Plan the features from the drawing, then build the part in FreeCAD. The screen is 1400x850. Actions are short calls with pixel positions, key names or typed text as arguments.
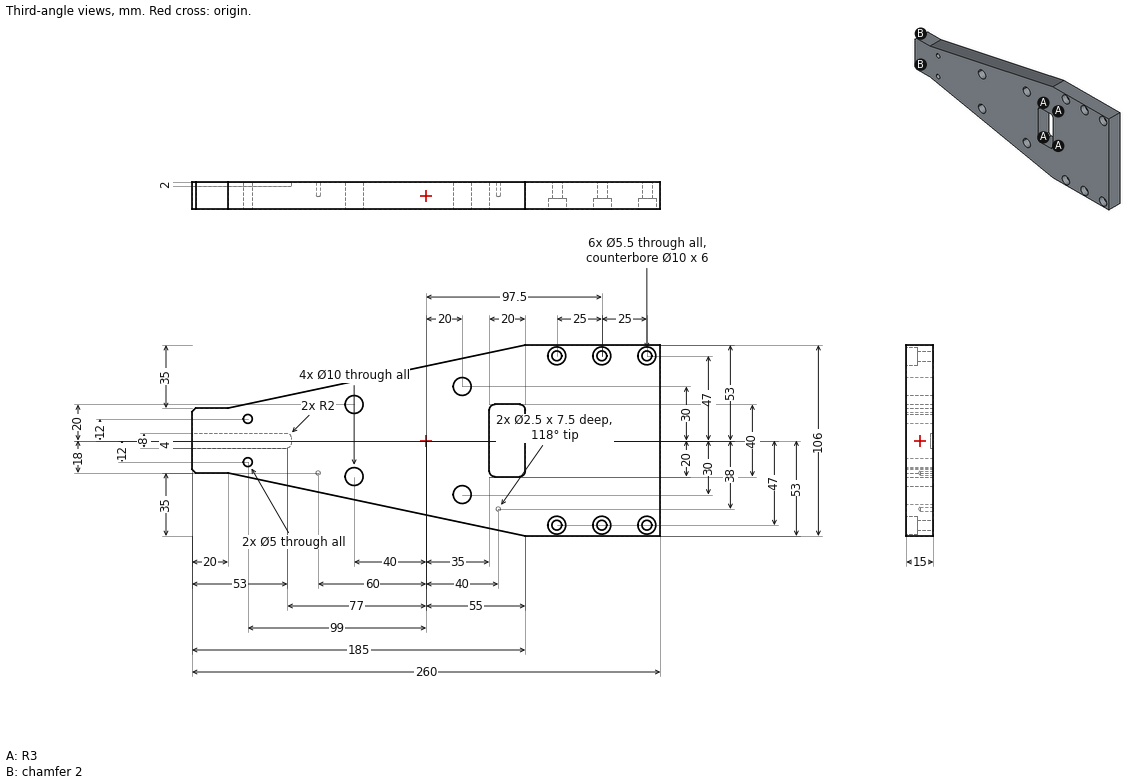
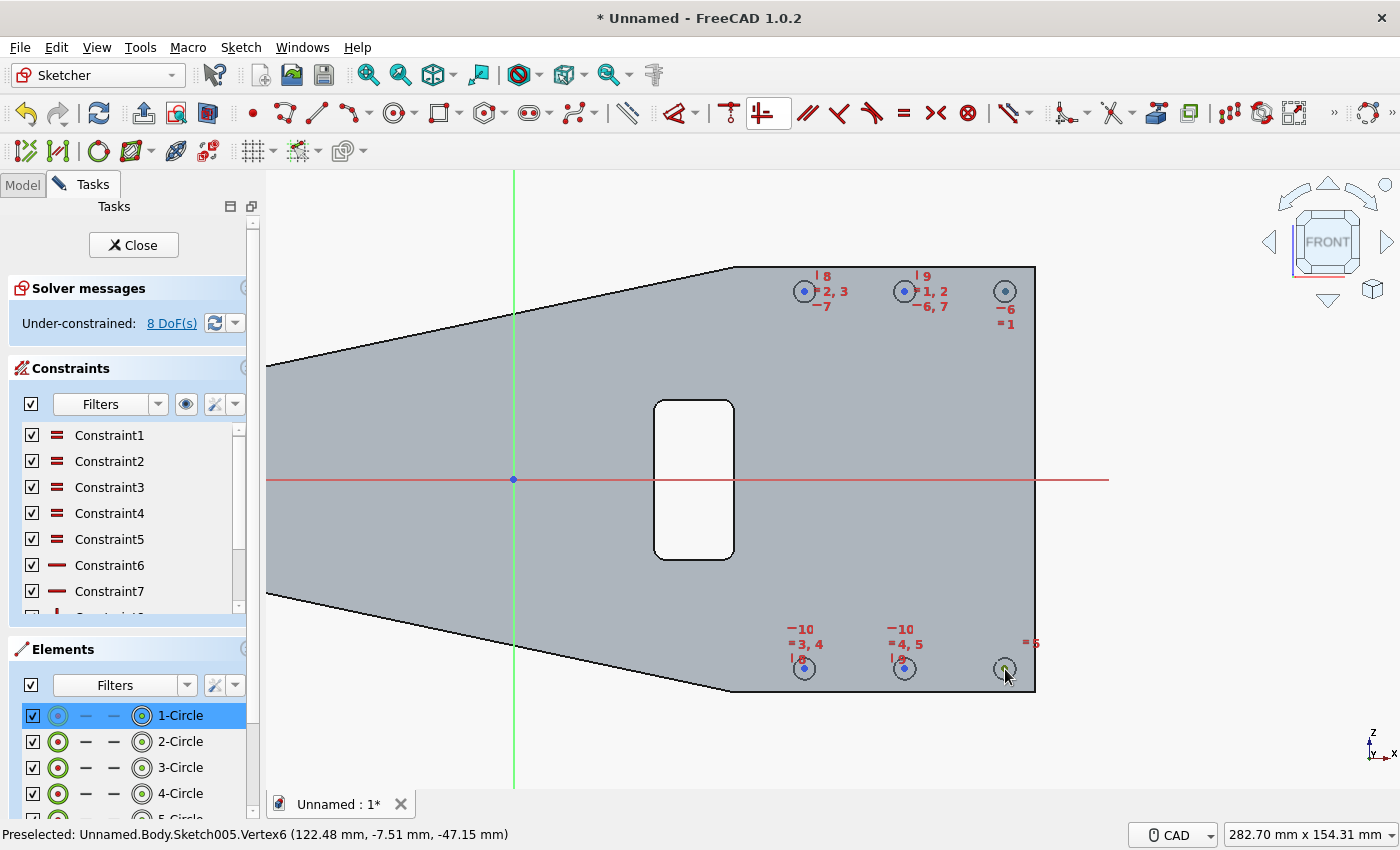
key(v)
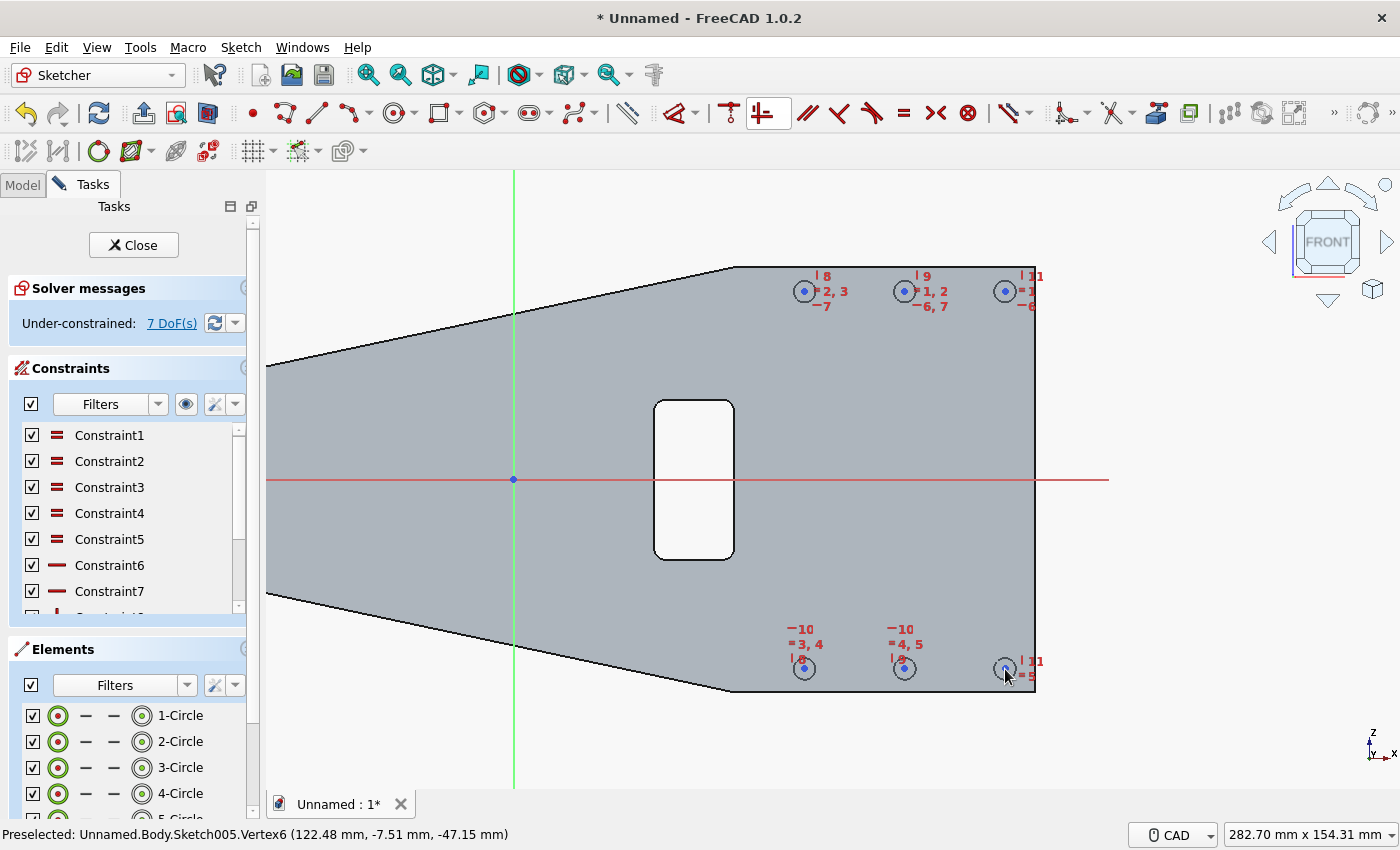
click(905, 669)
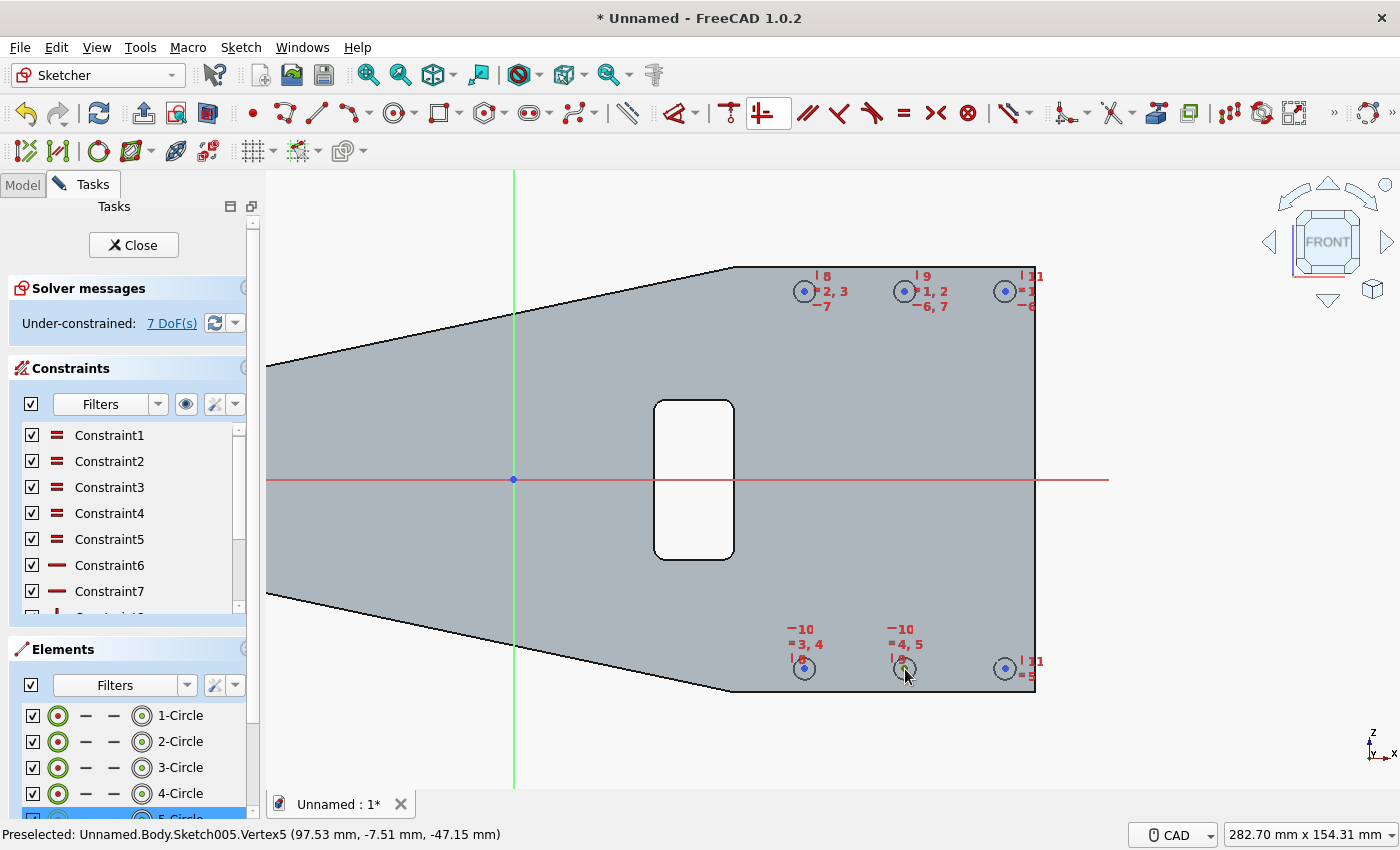
click(1005, 669)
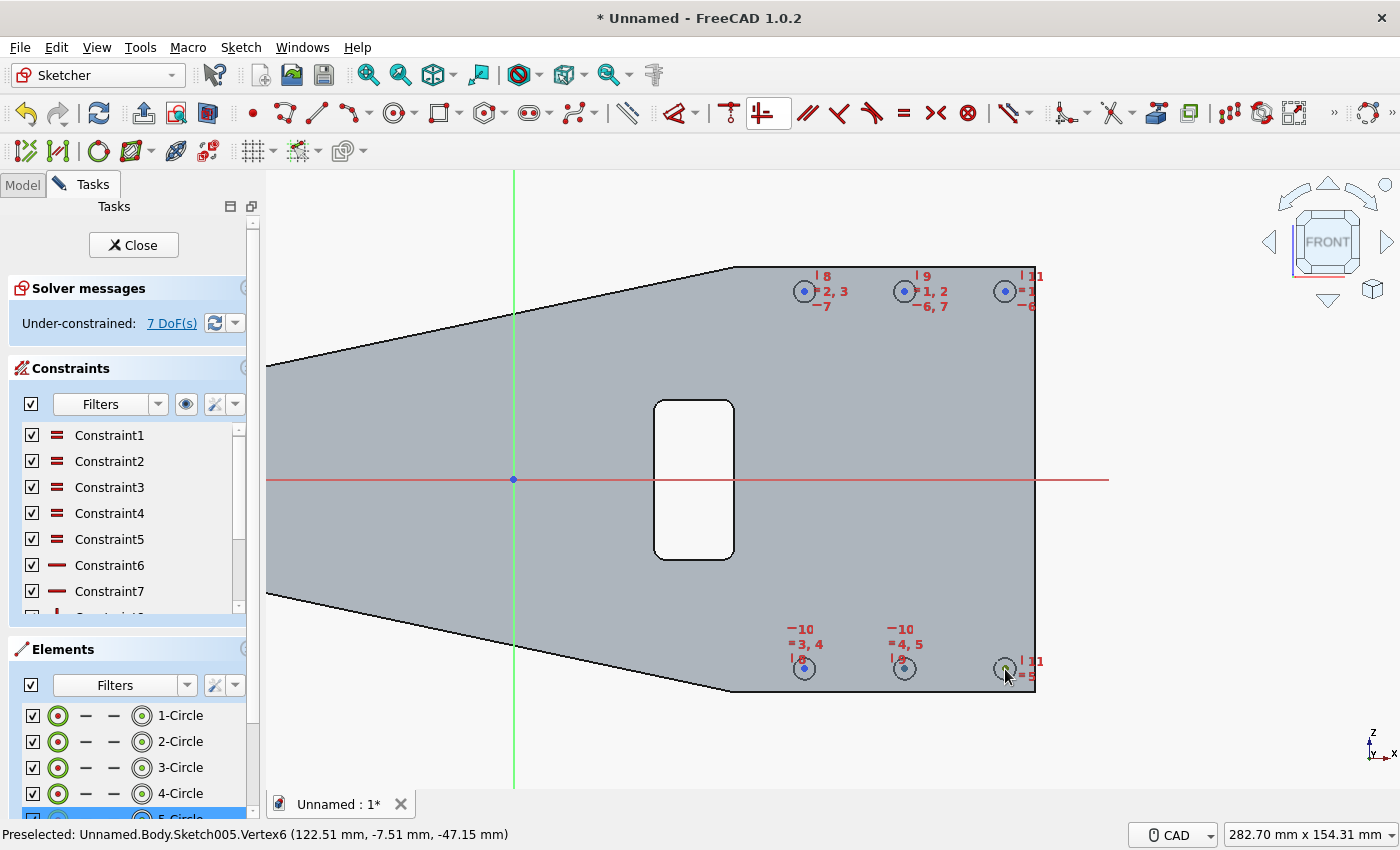
key(h)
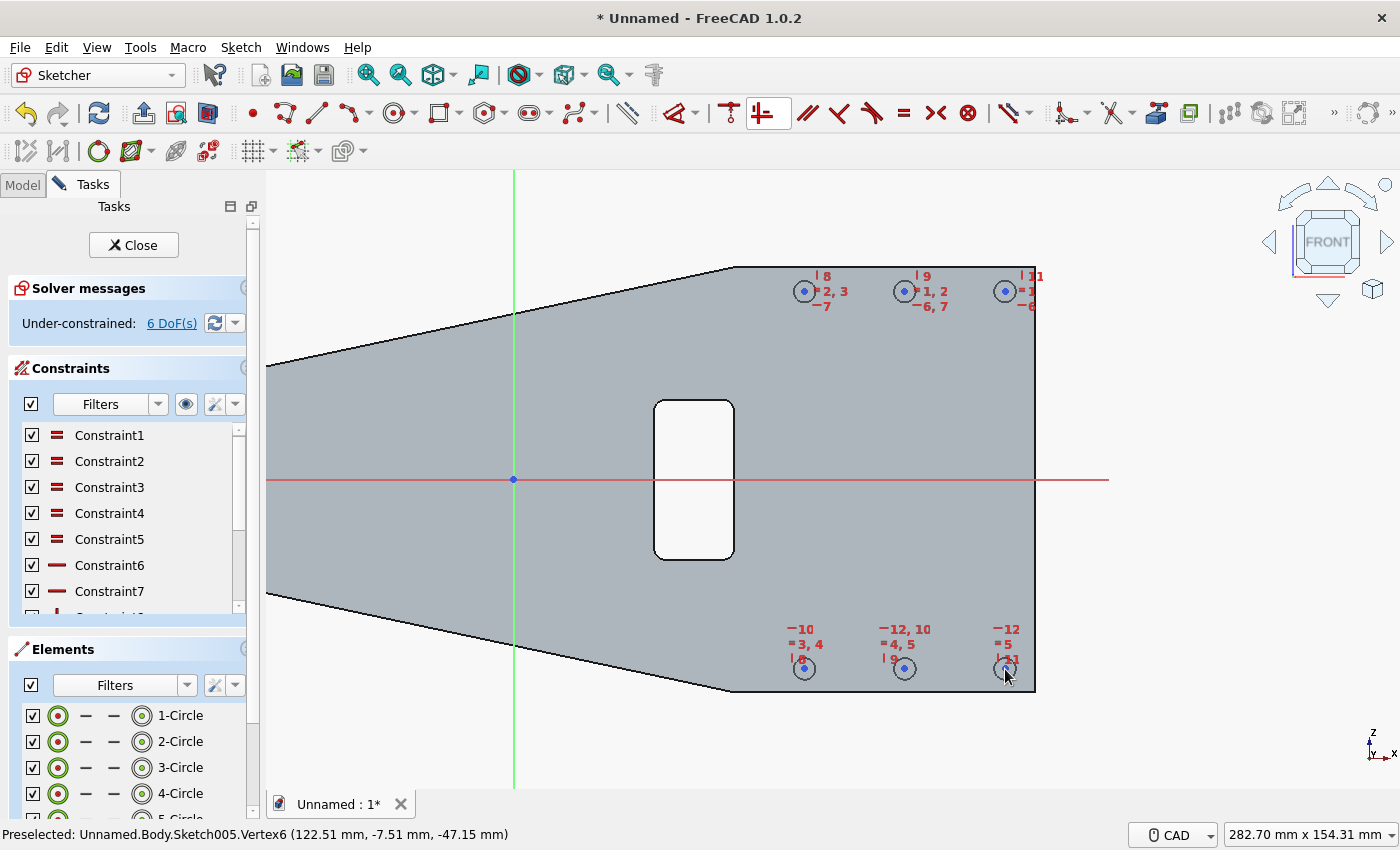
click(674, 114)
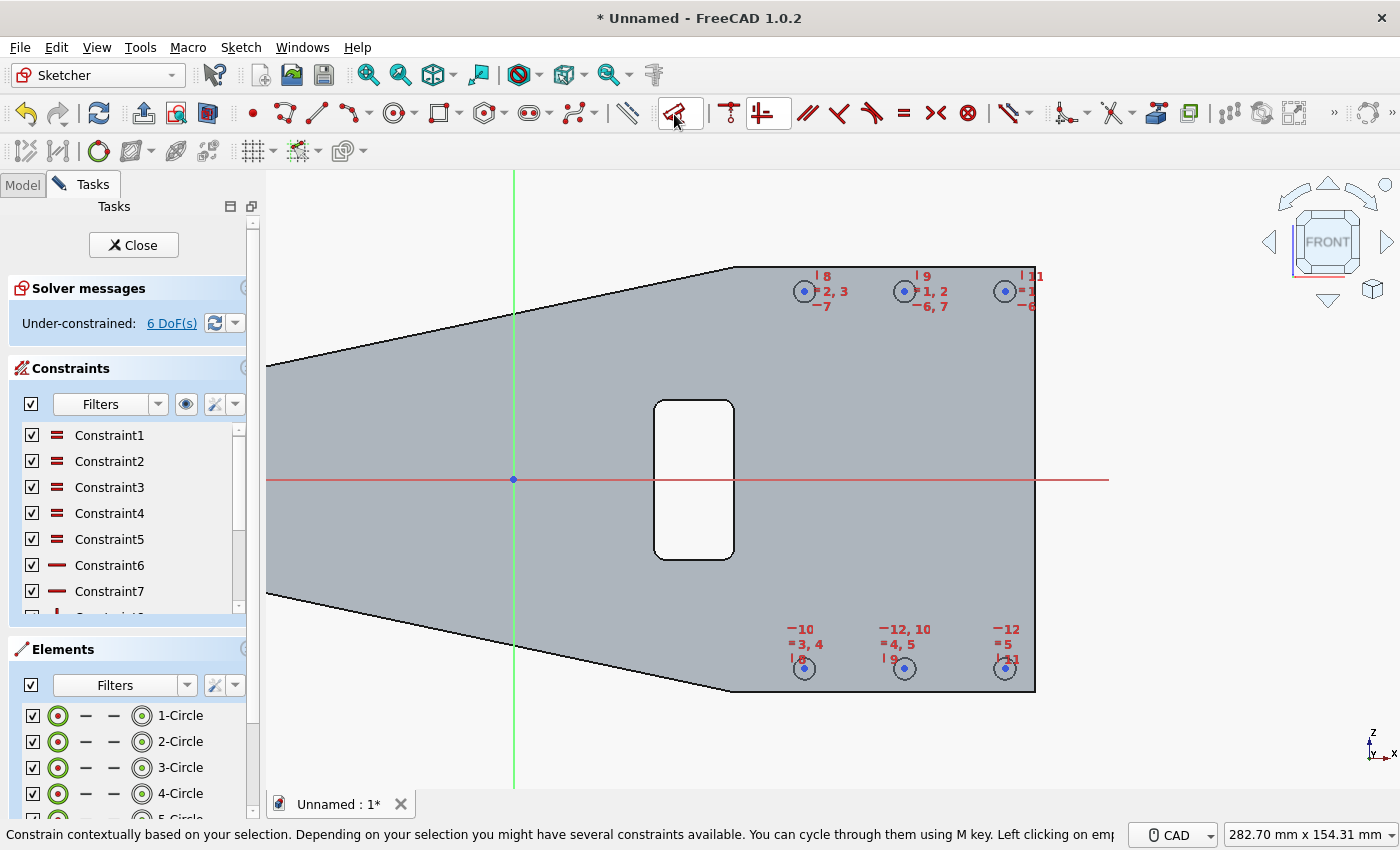
scroll(1013, 284, up, 3)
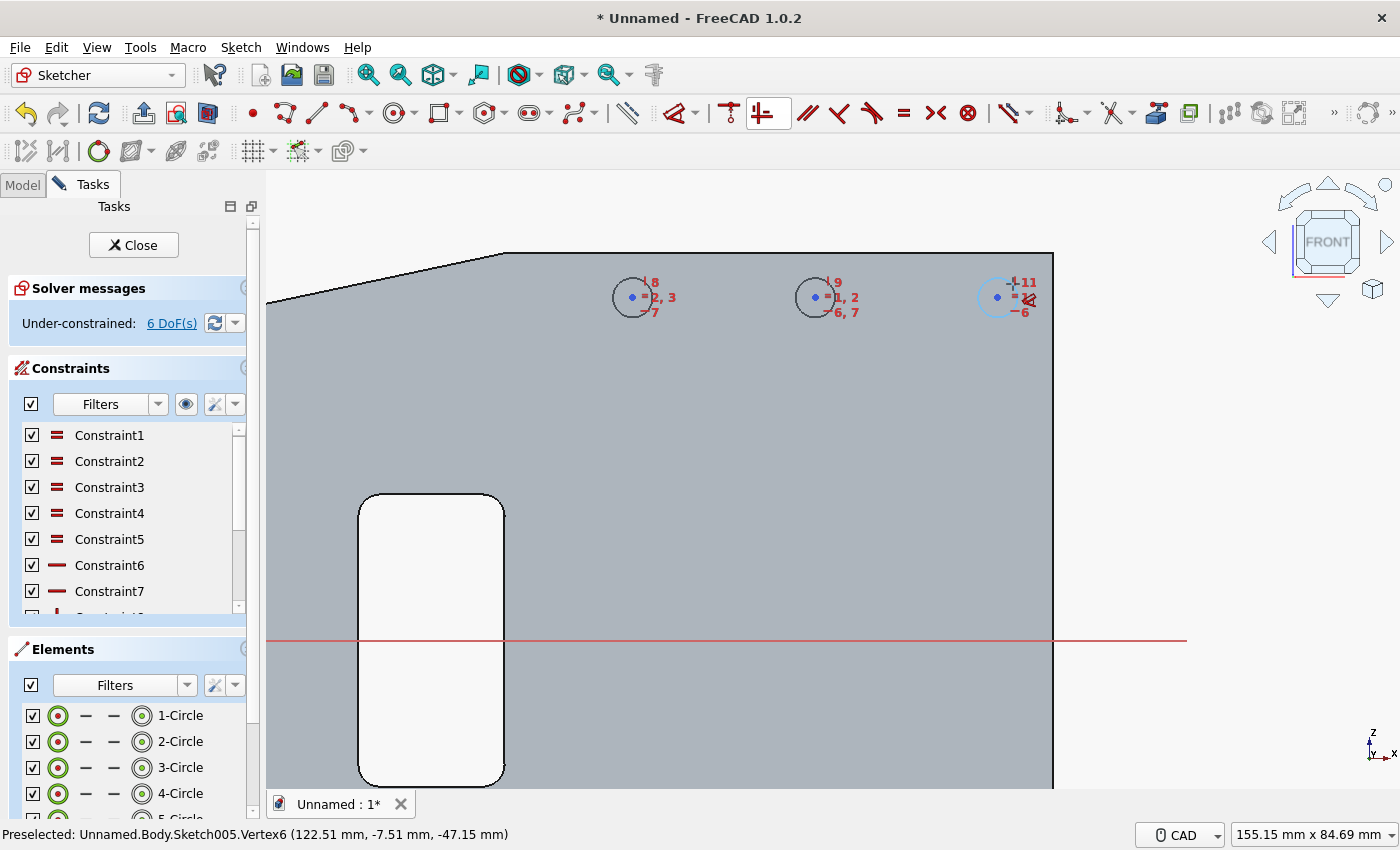
click(1012, 284)
click(1035, 262)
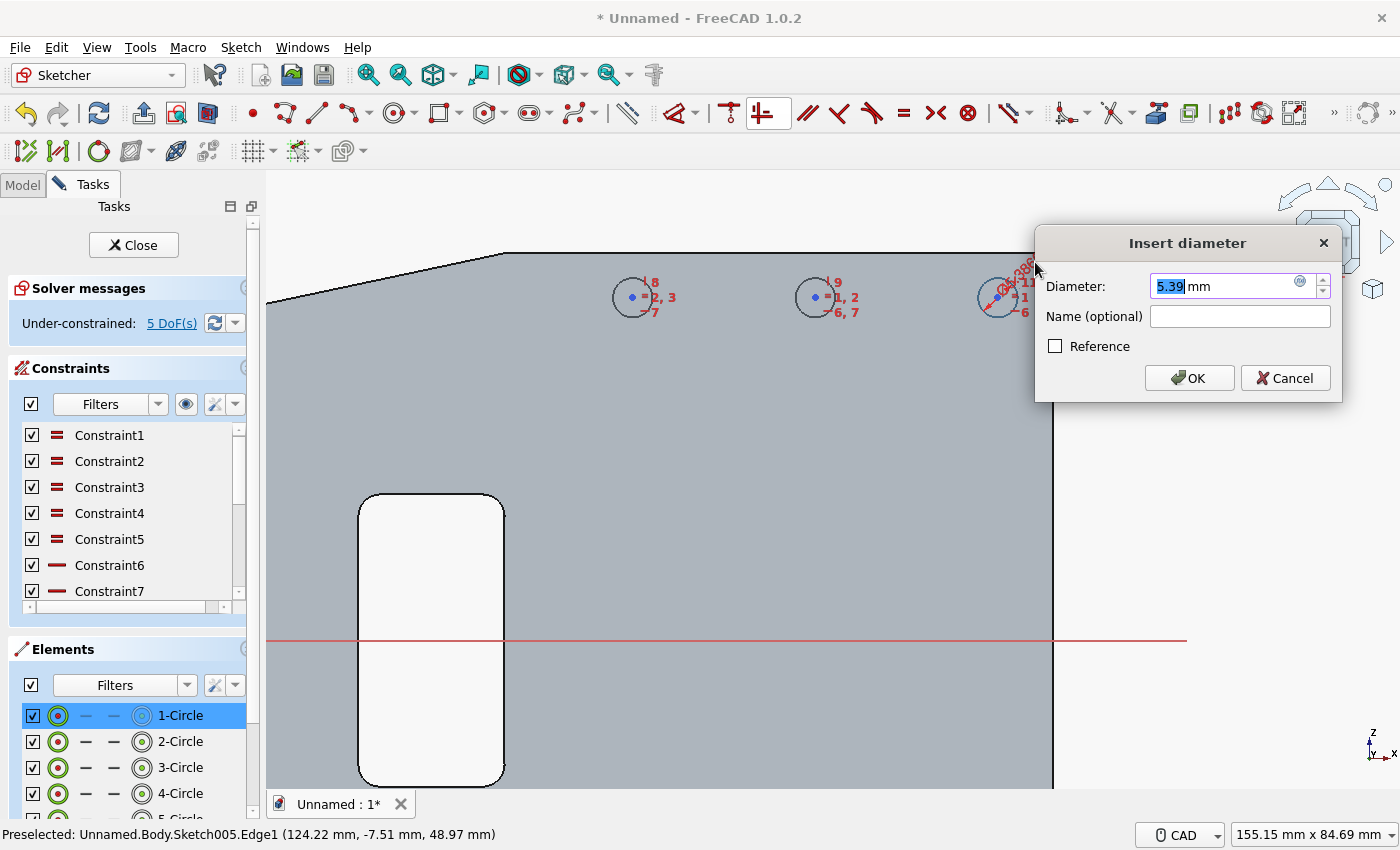
text(5.5)
key(Return)